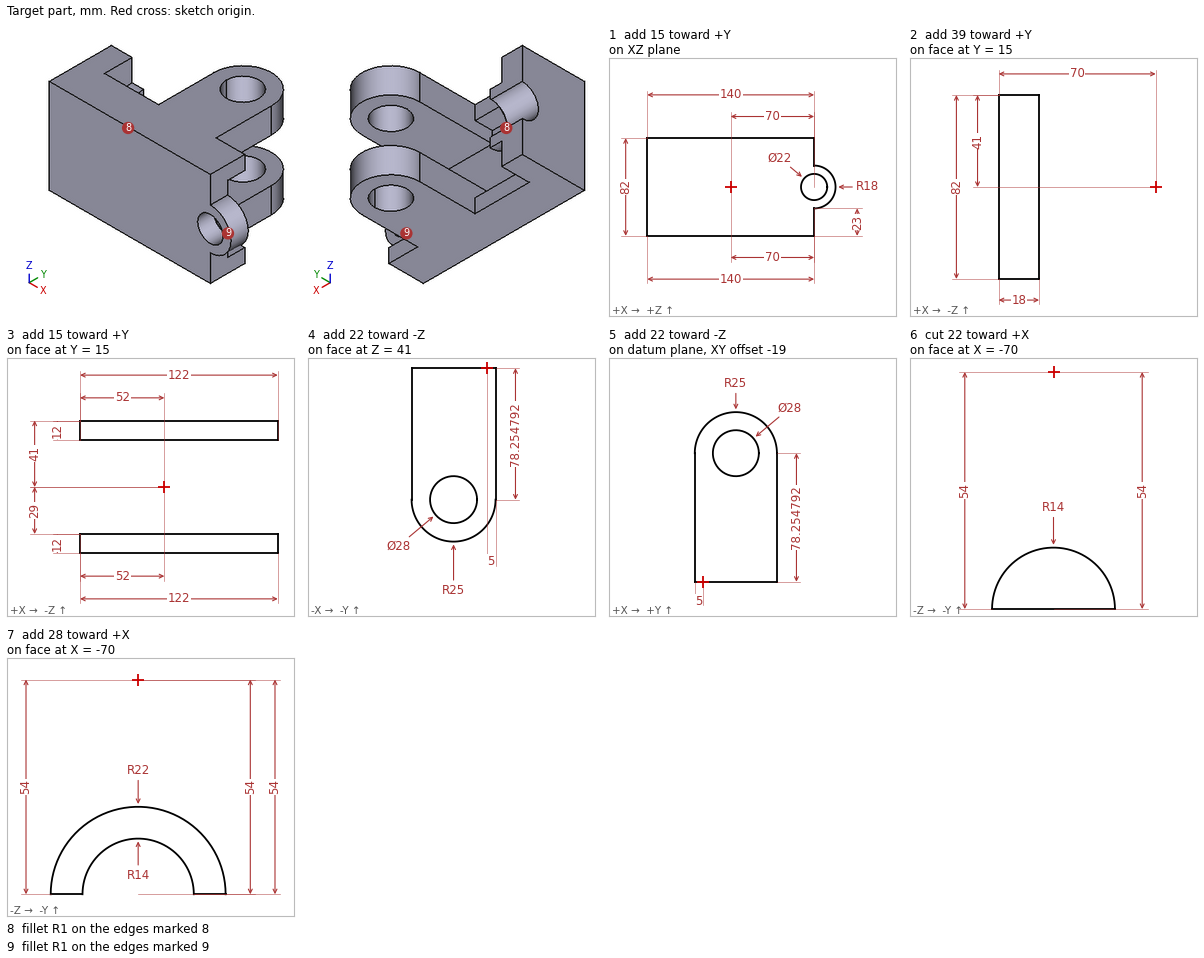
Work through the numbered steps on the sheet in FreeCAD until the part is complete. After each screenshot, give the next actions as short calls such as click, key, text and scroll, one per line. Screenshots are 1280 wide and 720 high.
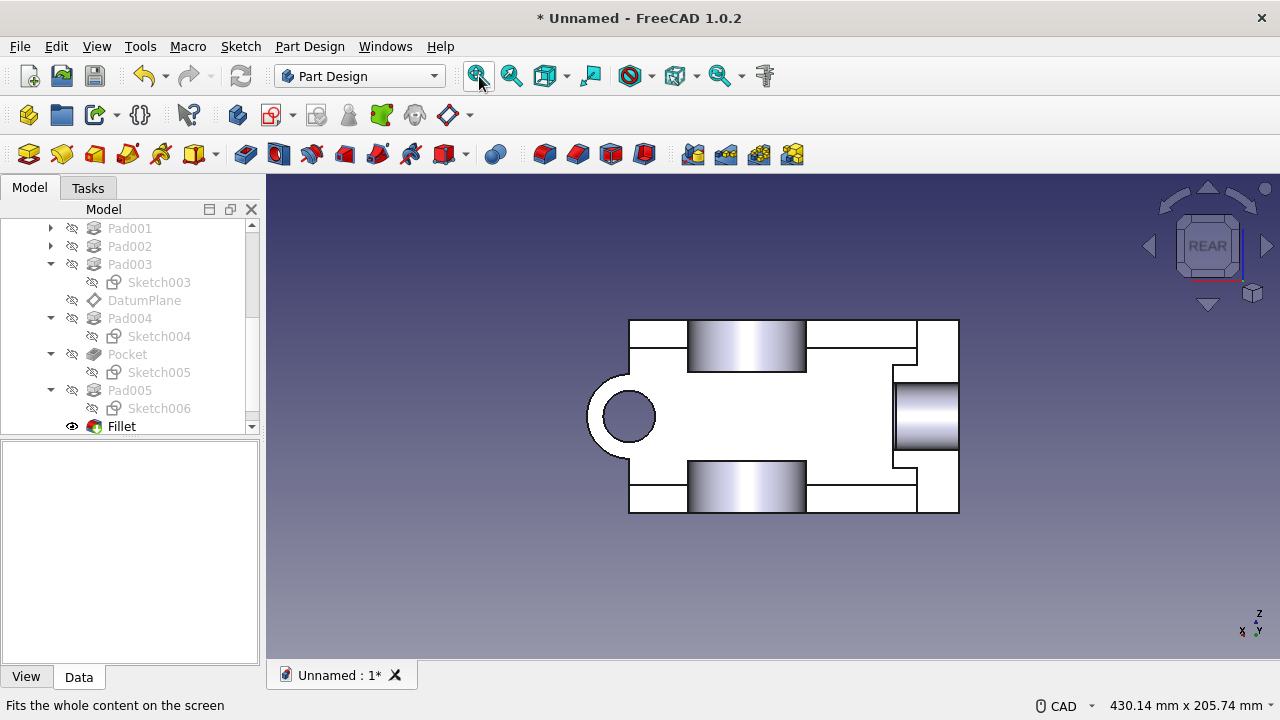
click(655, 416)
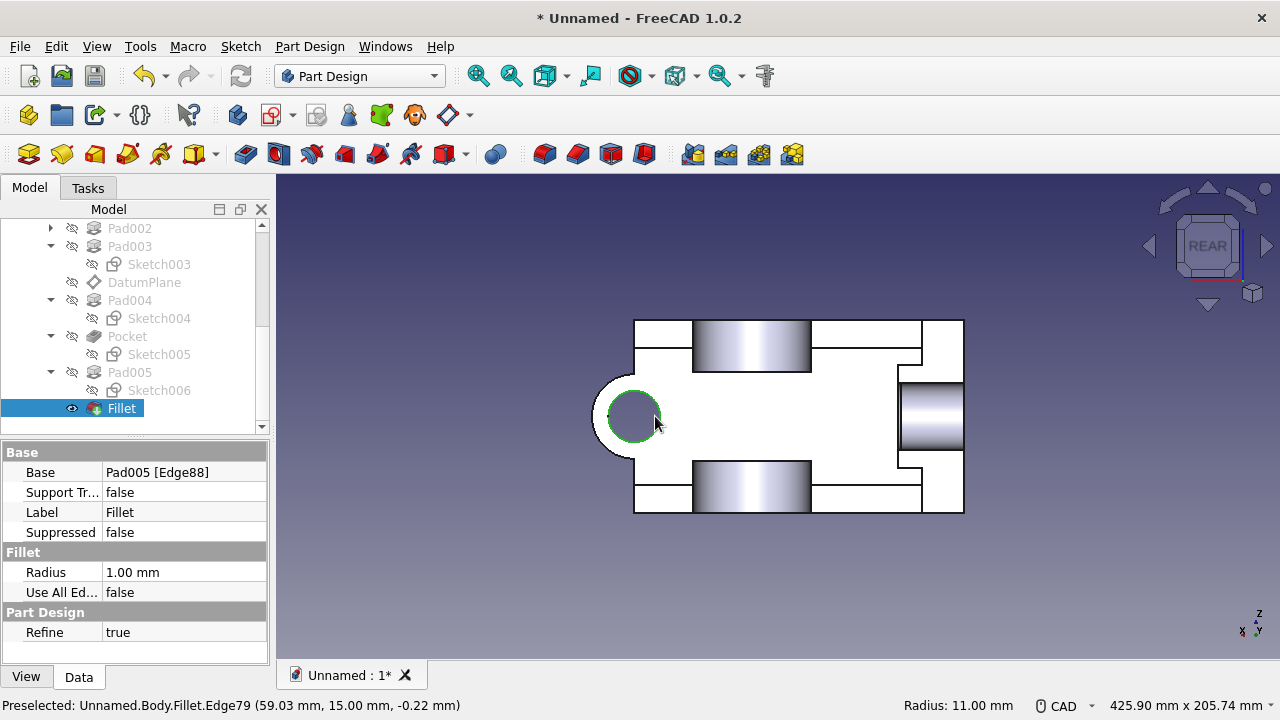
click(545, 154)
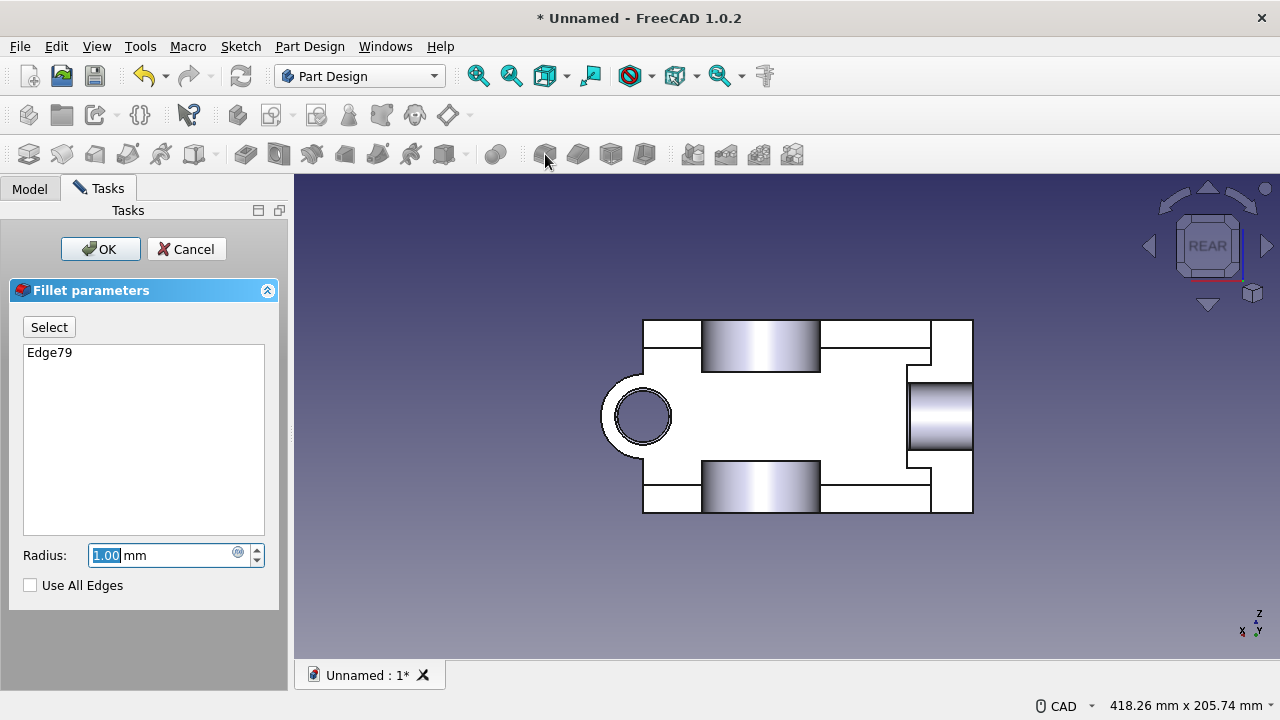
text(1)
key(Tab)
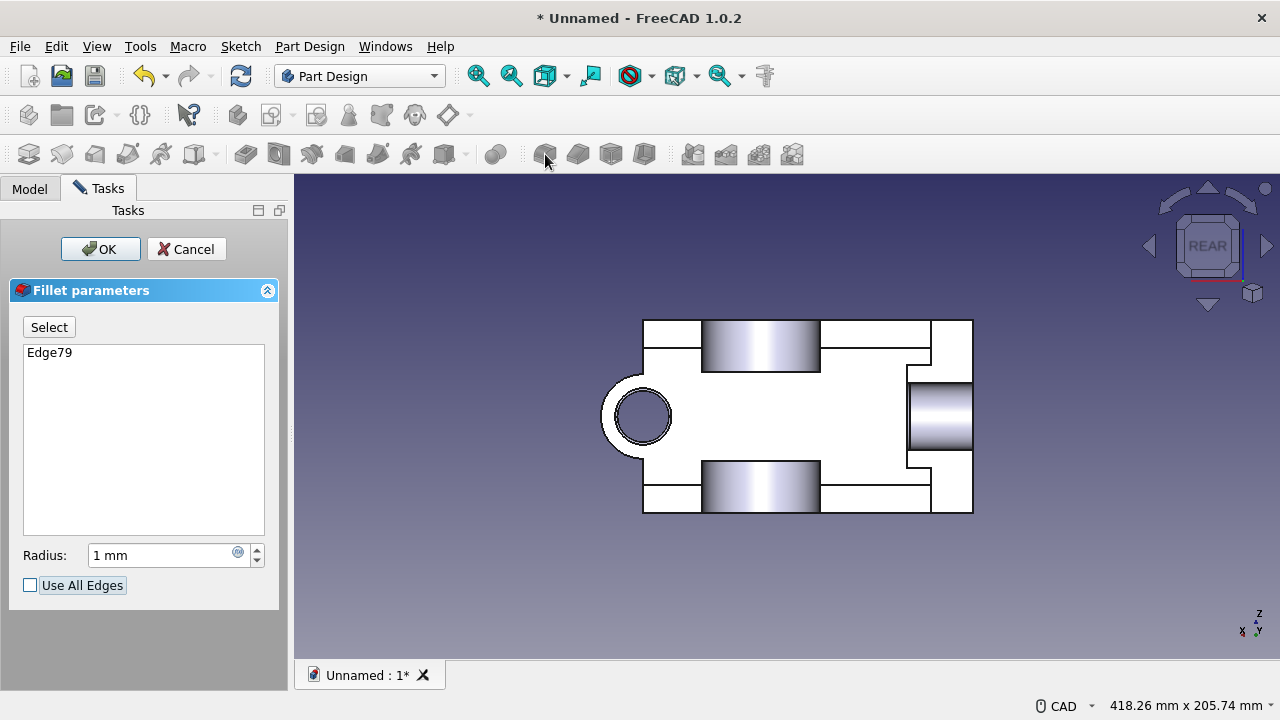
click(101, 249)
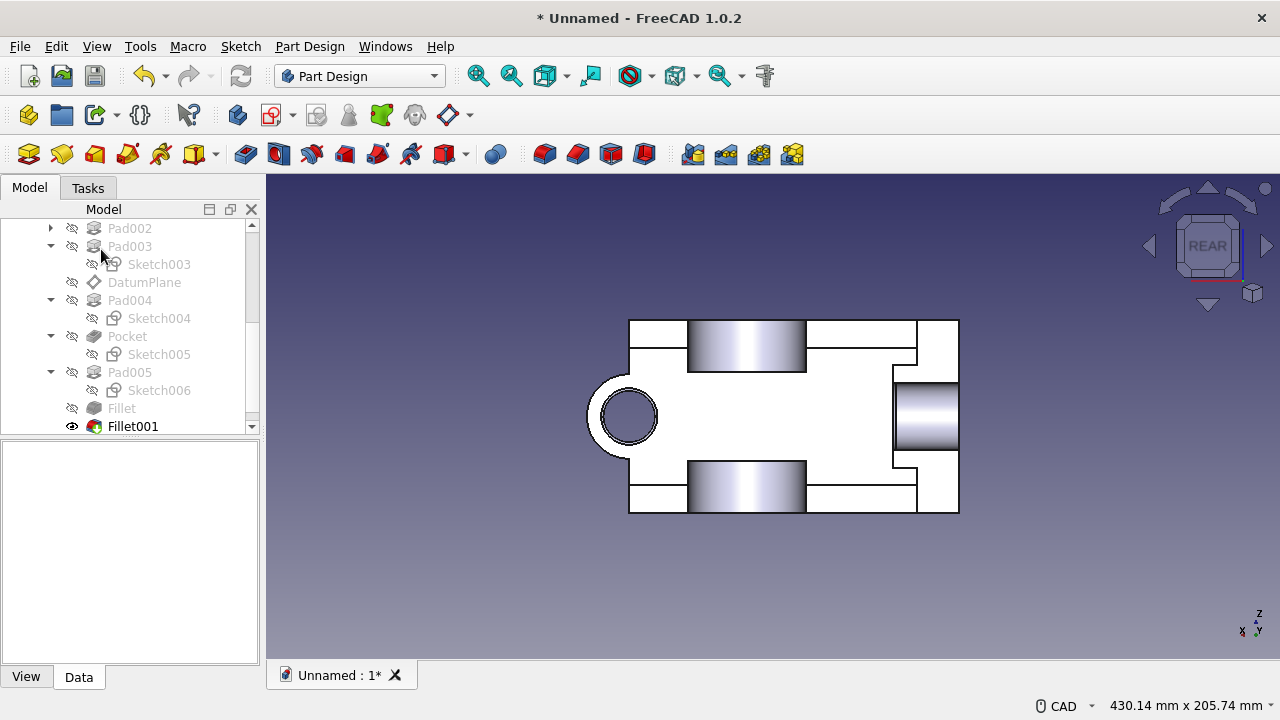
key(0)